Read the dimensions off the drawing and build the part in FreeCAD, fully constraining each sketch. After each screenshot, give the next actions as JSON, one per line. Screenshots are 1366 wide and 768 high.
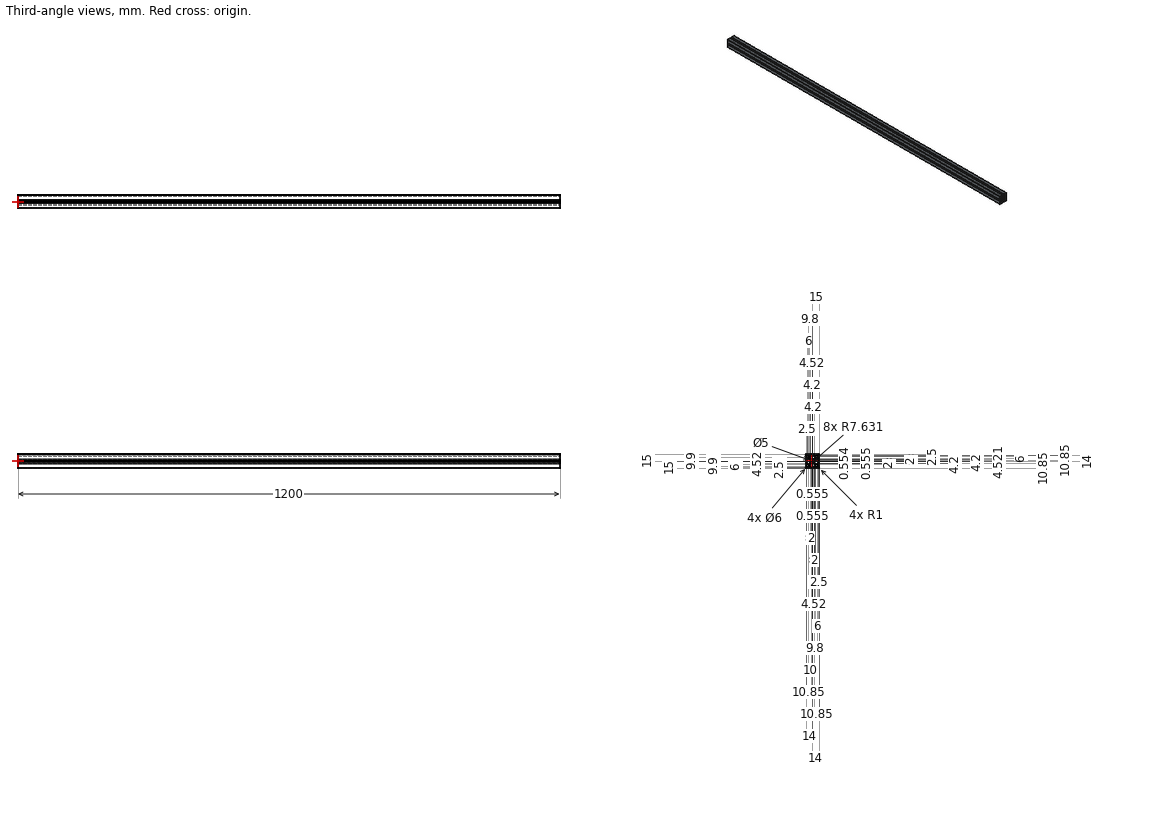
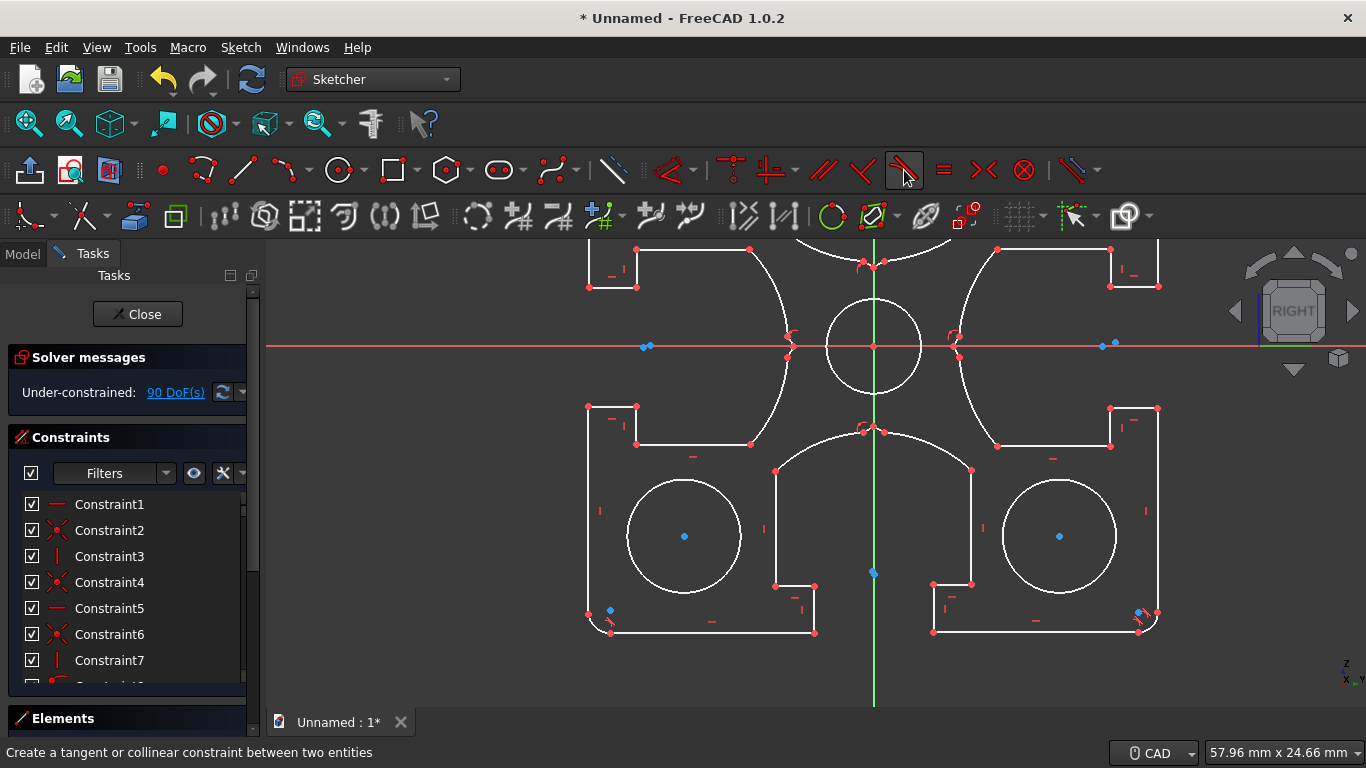
{"action": "scroll", "coordinate": [594, 627], "scroll_direction": "down", "scroll_amount": 3}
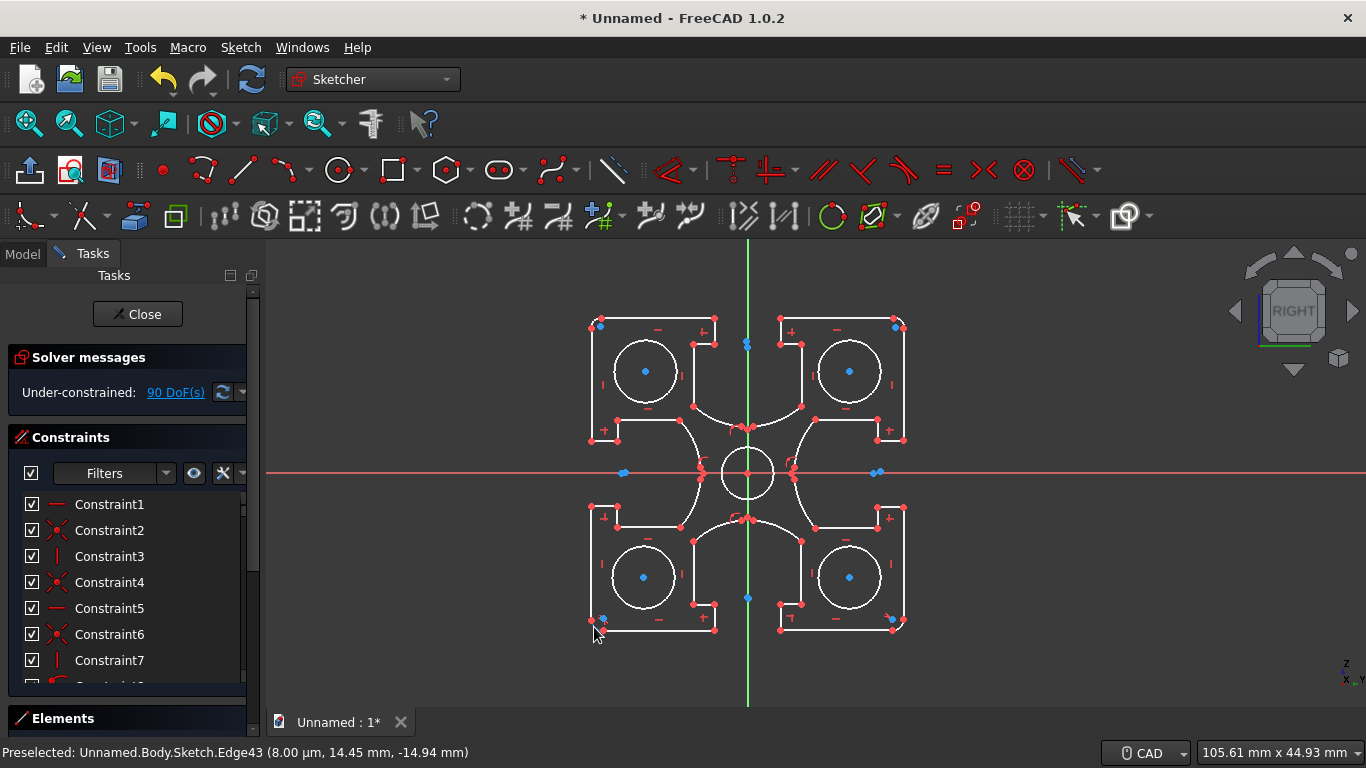
{"action": "left_click", "coordinate": [904, 407]}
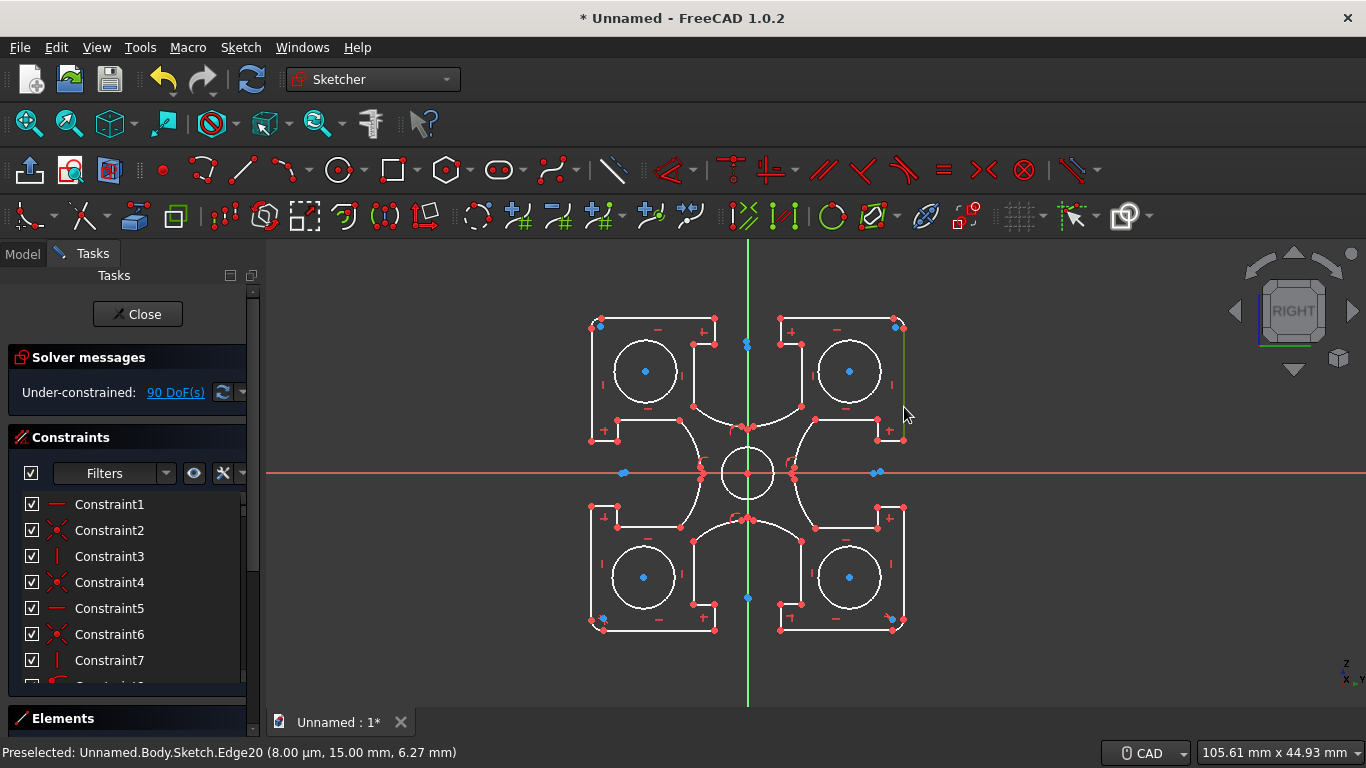
{"action": "scroll", "coordinate": [901, 321], "scroll_direction": "up", "scroll_amount": 3}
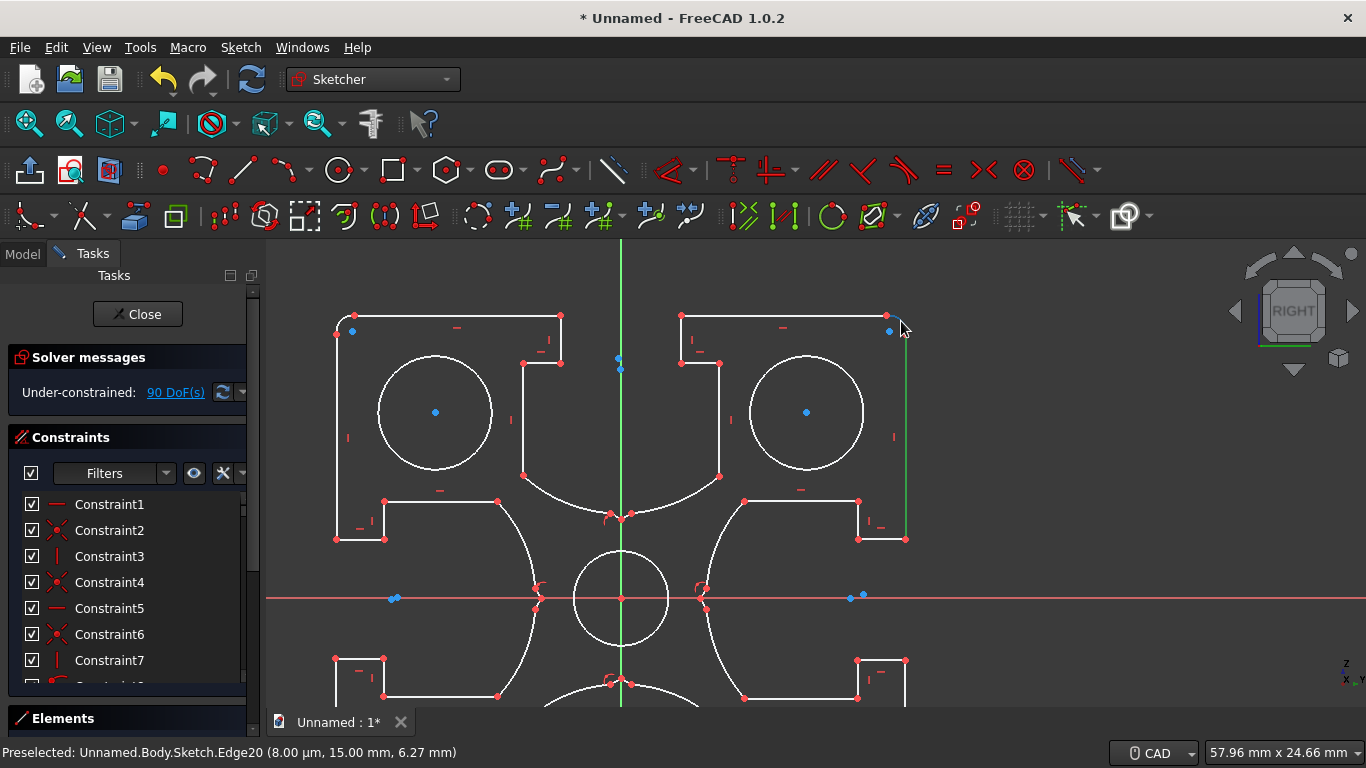
{"action": "left_click", "coordinate": [901, 320]}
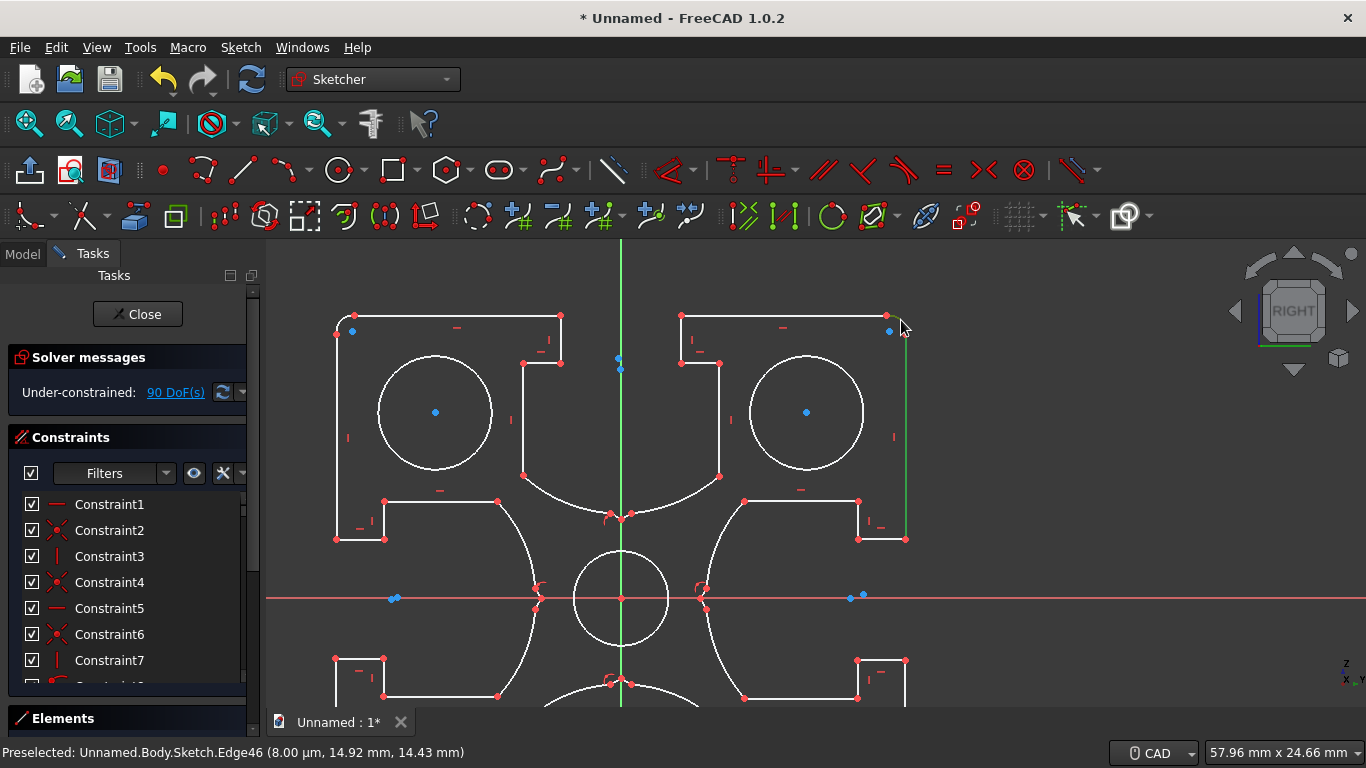
{"action": "left_click", "coordinate": [904, 170]}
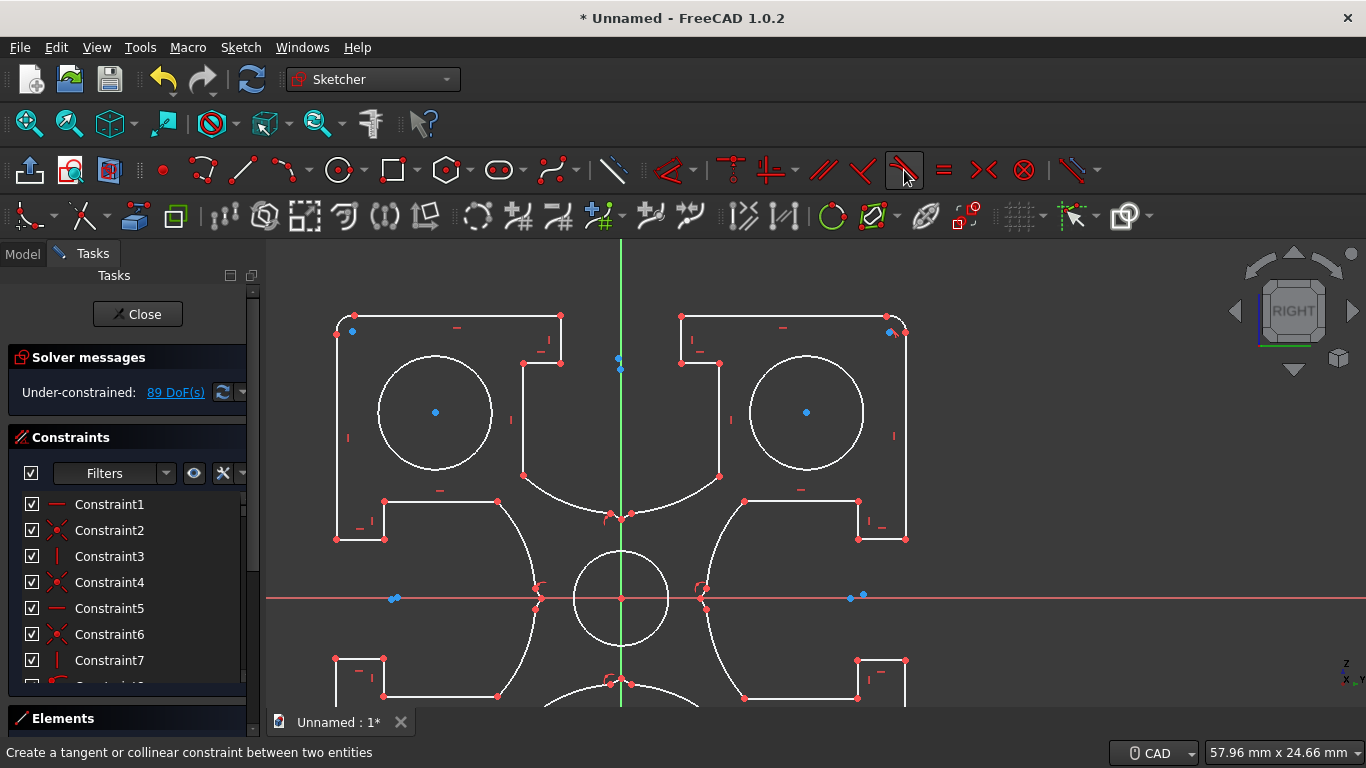
{"action": "left_click", "coordinate": [825, 316]}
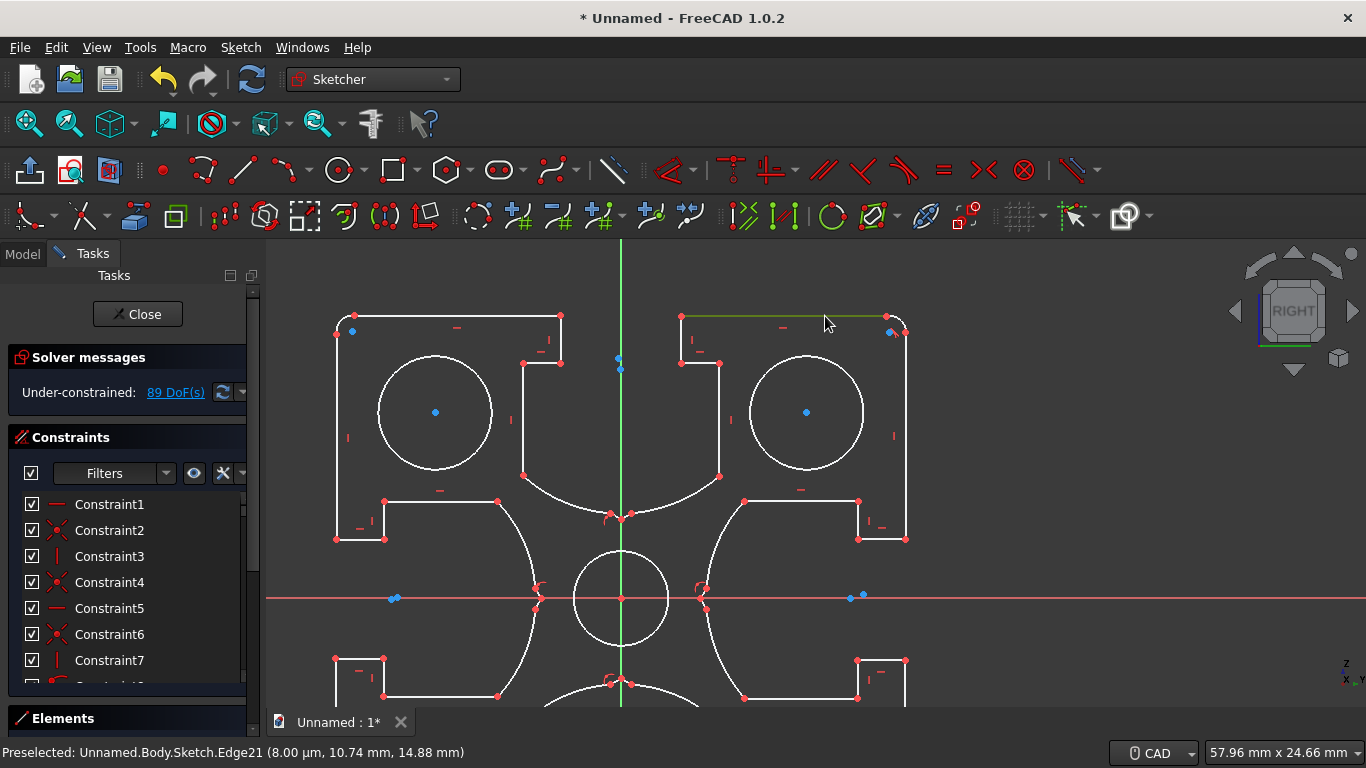
{"action": "left_click", "coordinate": [900, 320]}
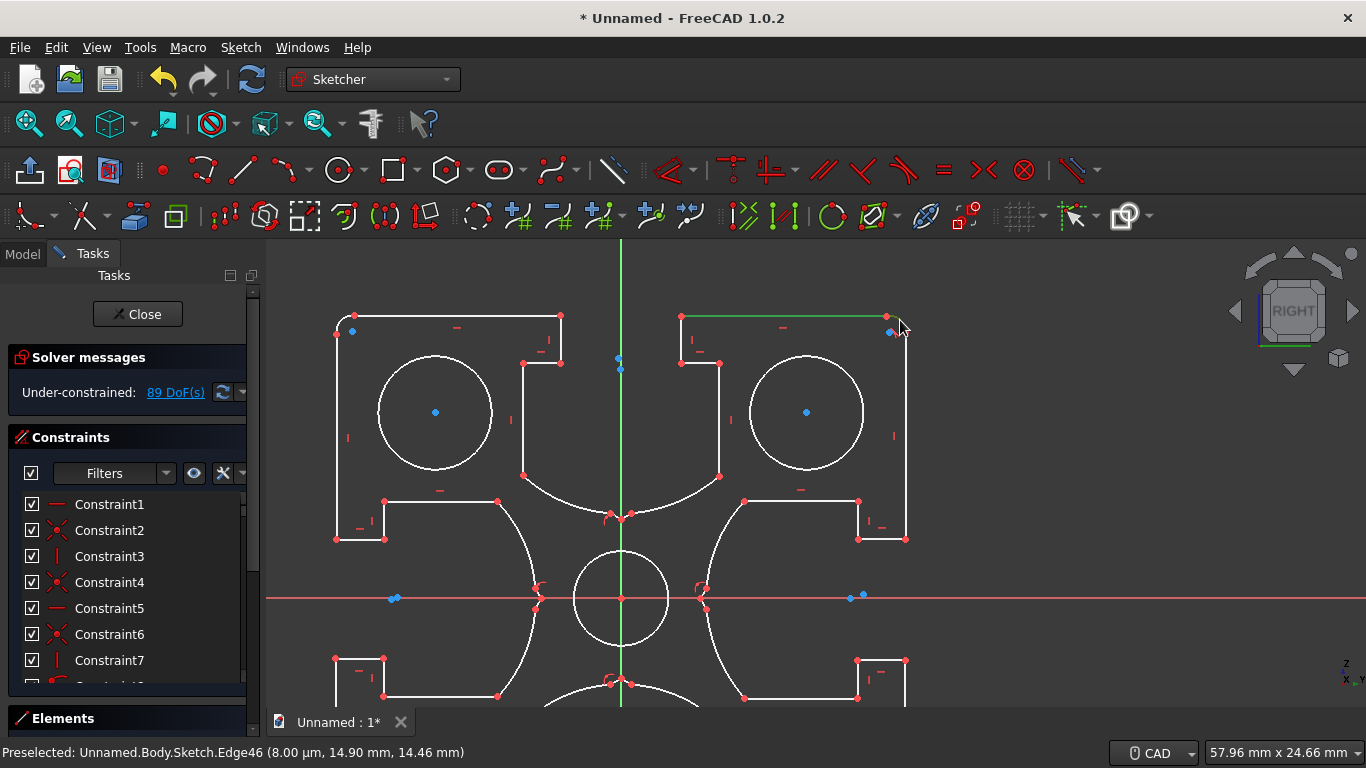
{"action": "left_click", "coordinate": [904, 170]}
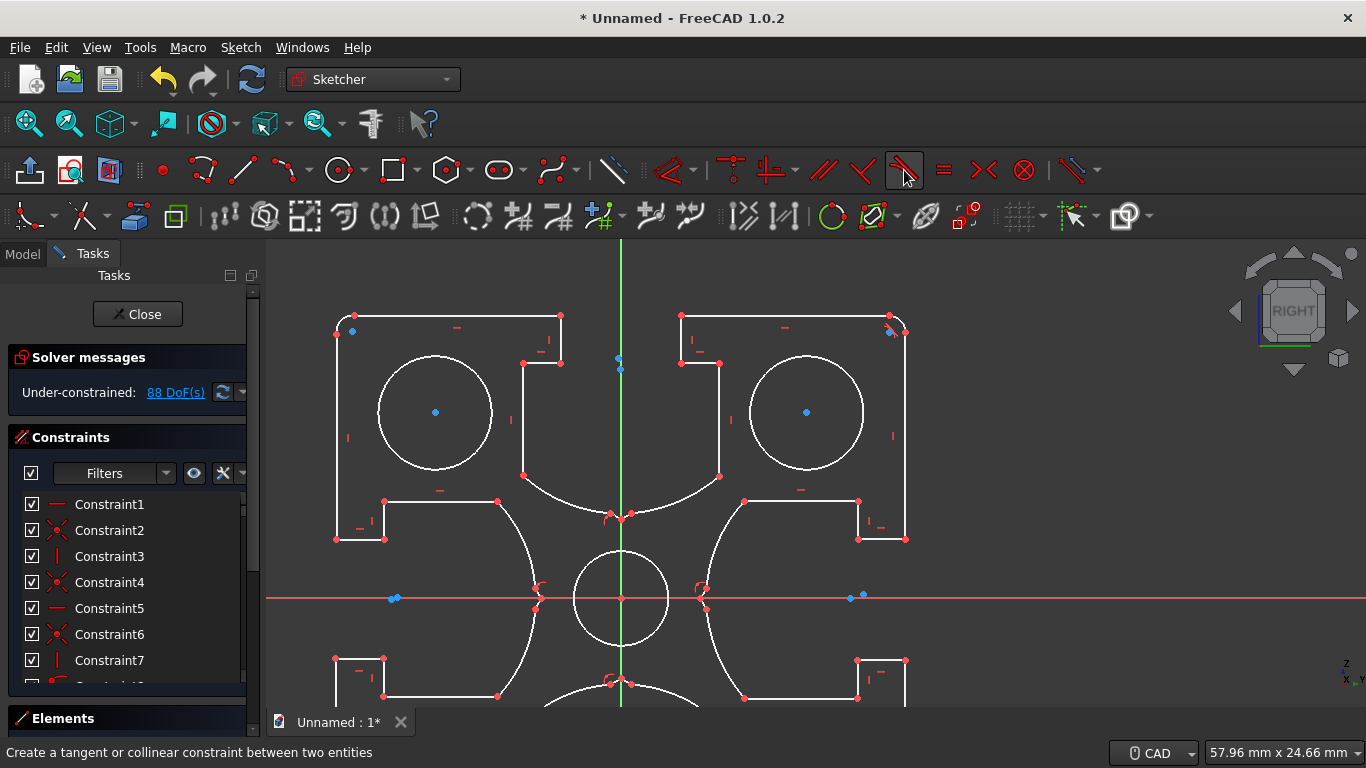
{"action": "left_click", "coordinate": [499, 316]}